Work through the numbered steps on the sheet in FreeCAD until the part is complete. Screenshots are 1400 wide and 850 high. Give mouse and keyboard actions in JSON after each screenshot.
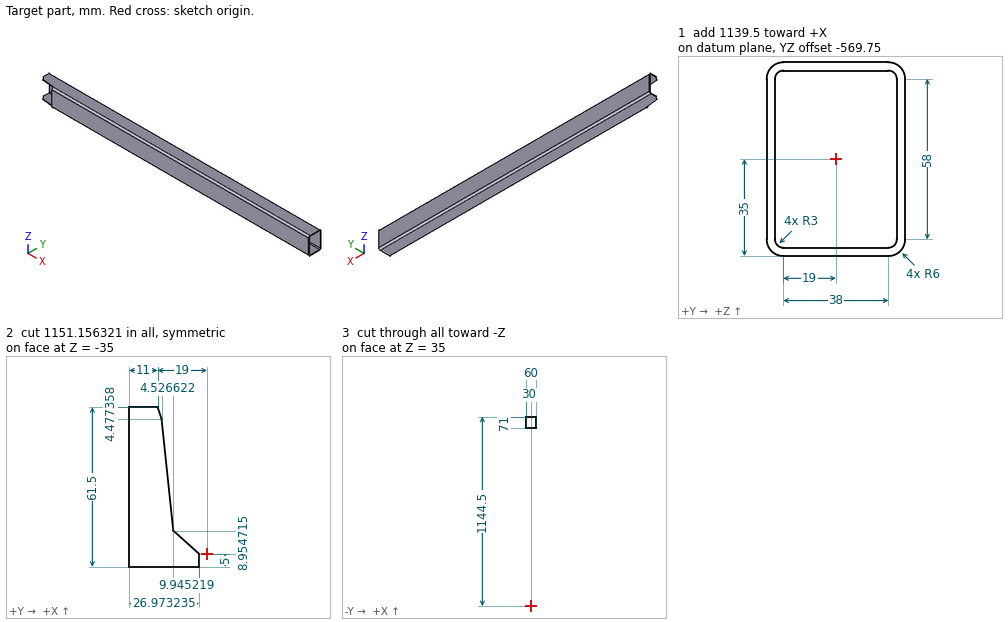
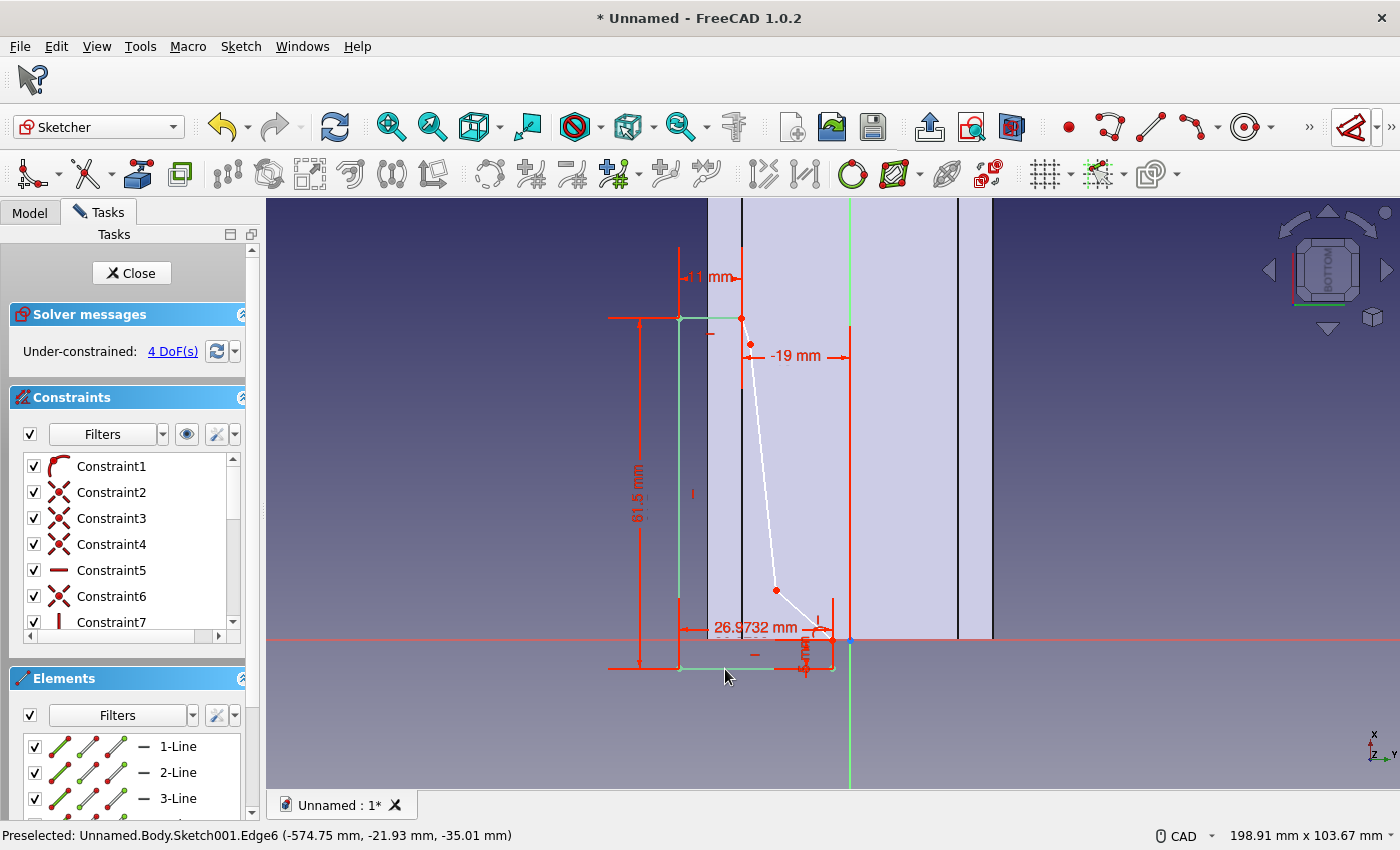
{"action": "left_click", "coordinate": [776, 590]}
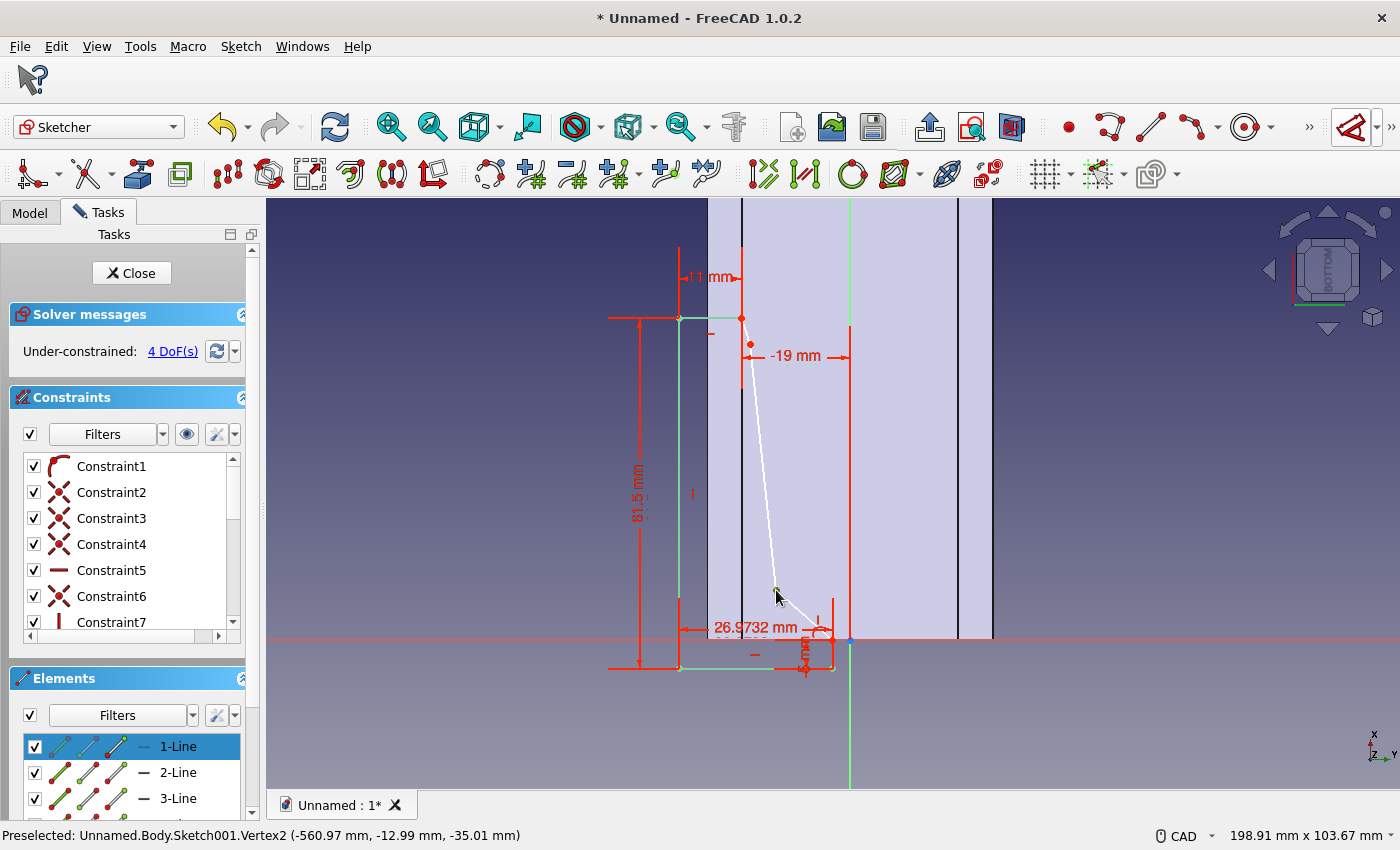
{"action": "key", "text": "i"}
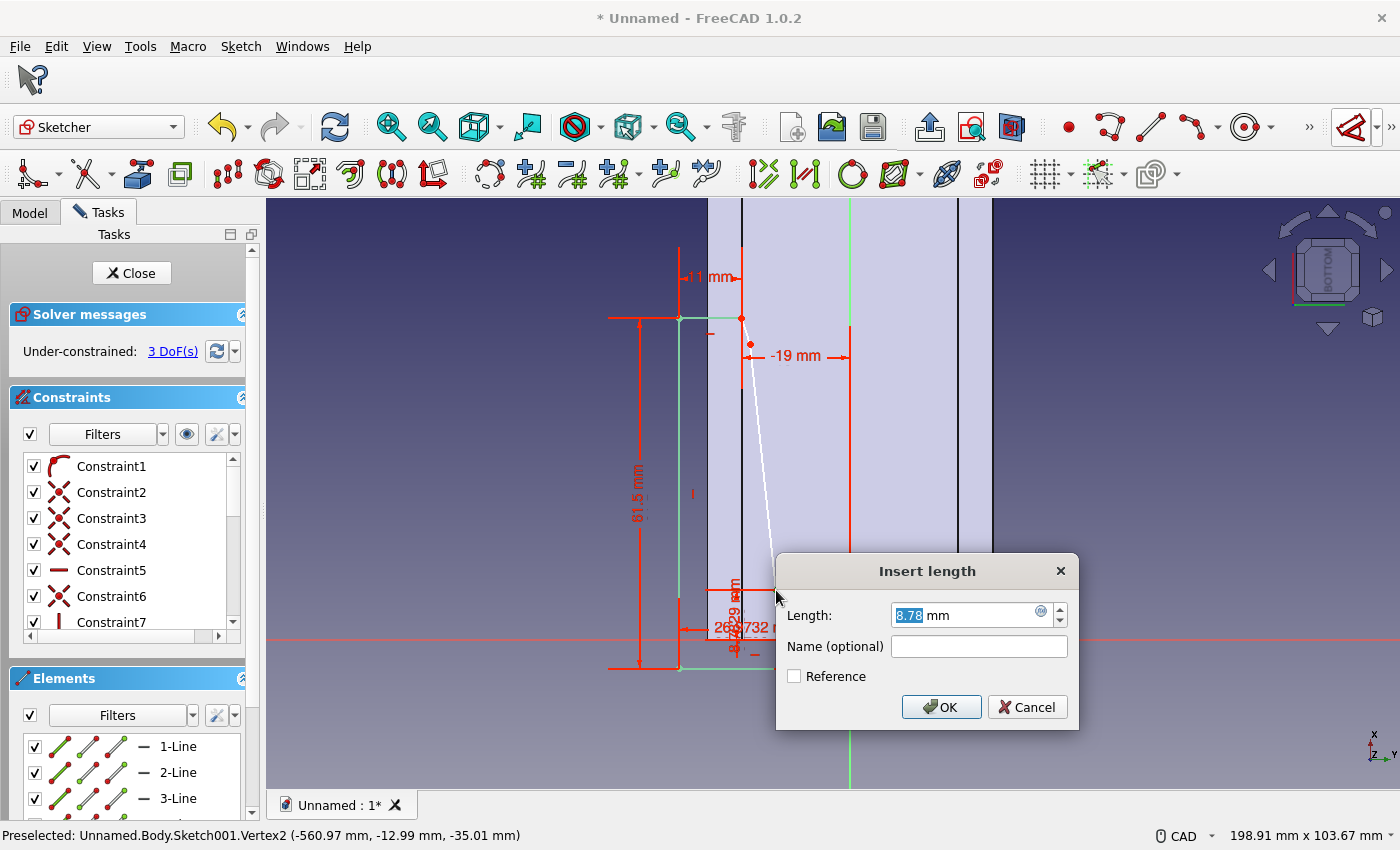
{"action": "type", "text": "8.954715"}
{"action": "key", "text": "Return"}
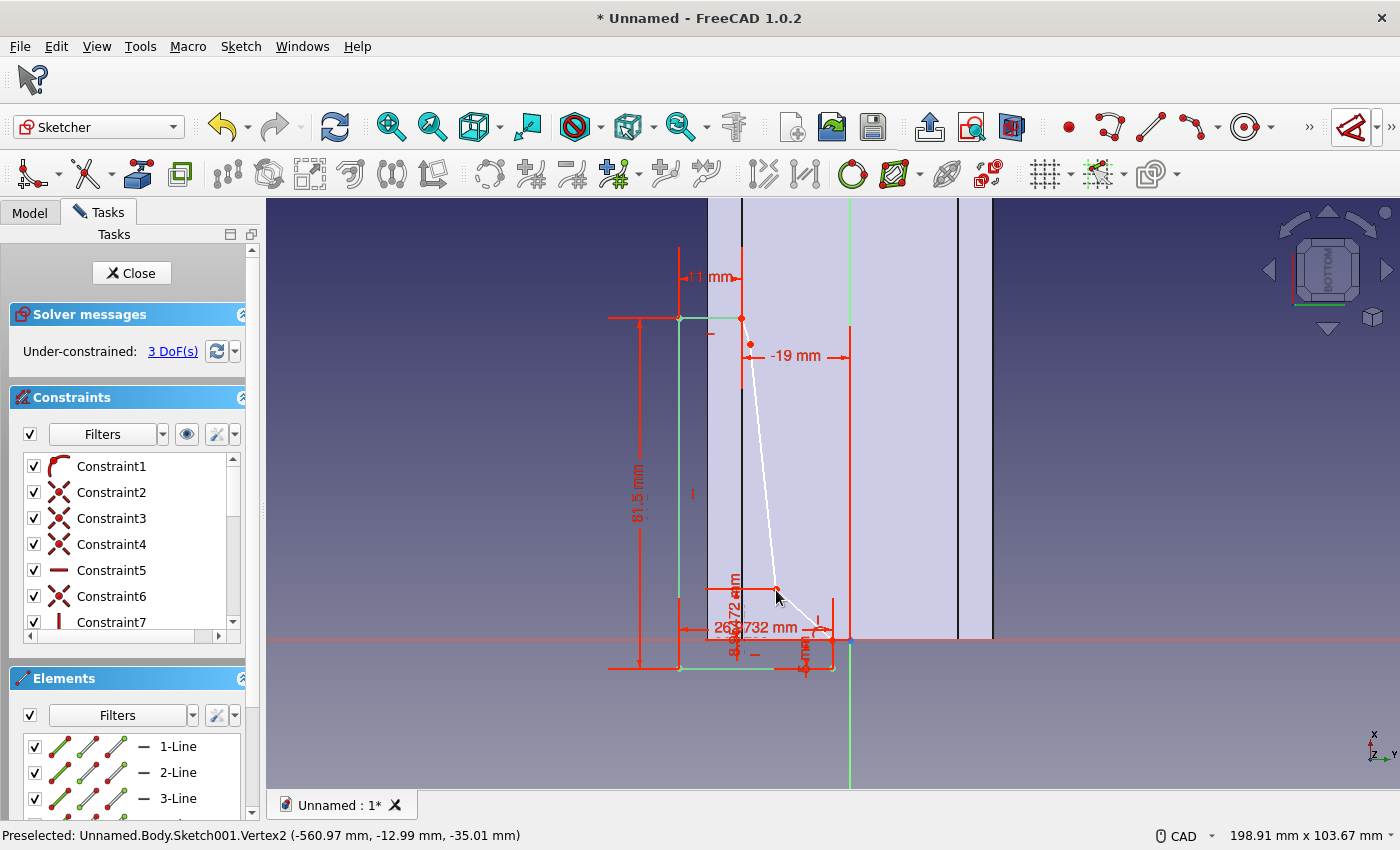
{"action": "left_click", "coordinate": [793, 605]}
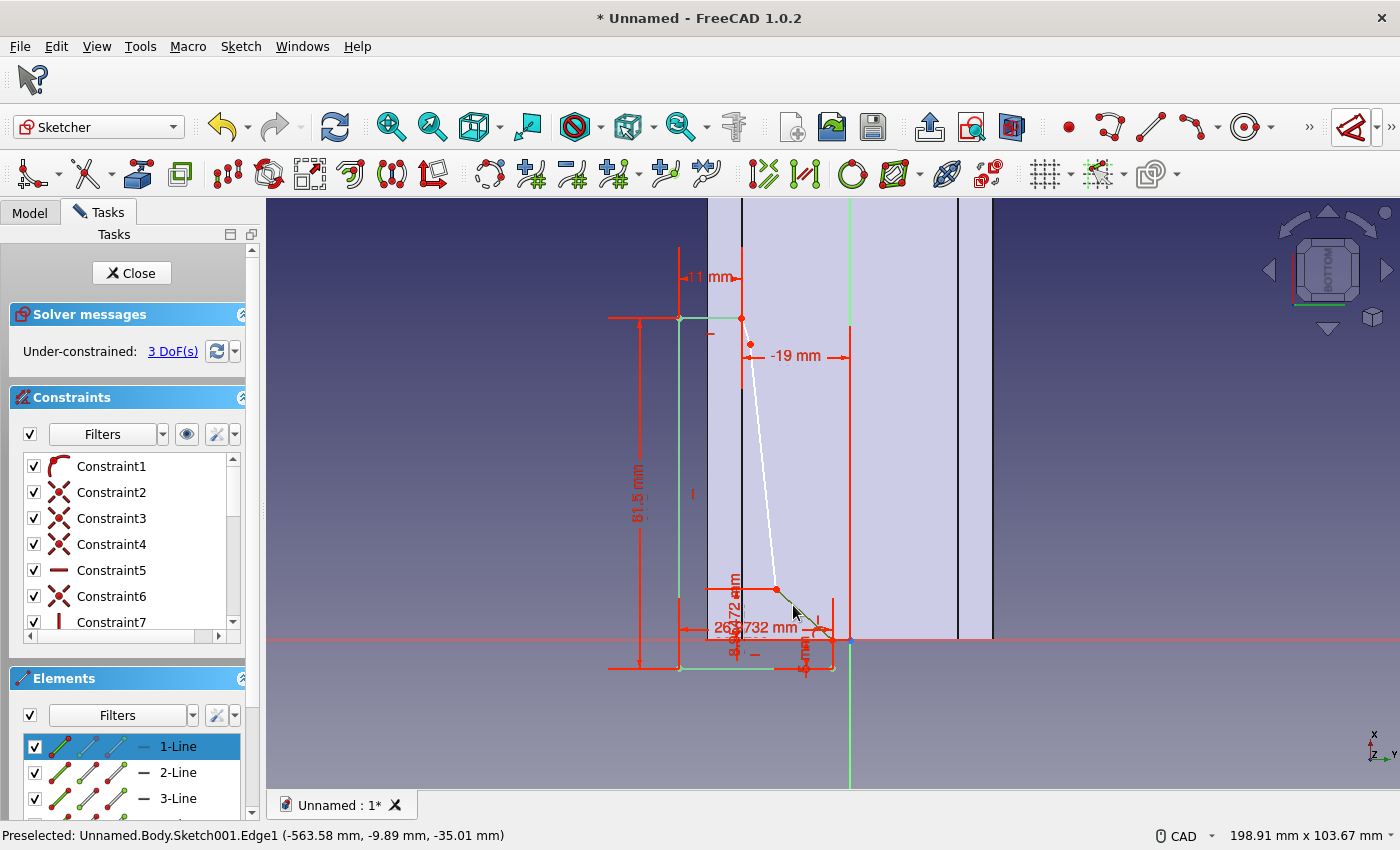
{"action": "left_click", "coordinate": [1376, 128]}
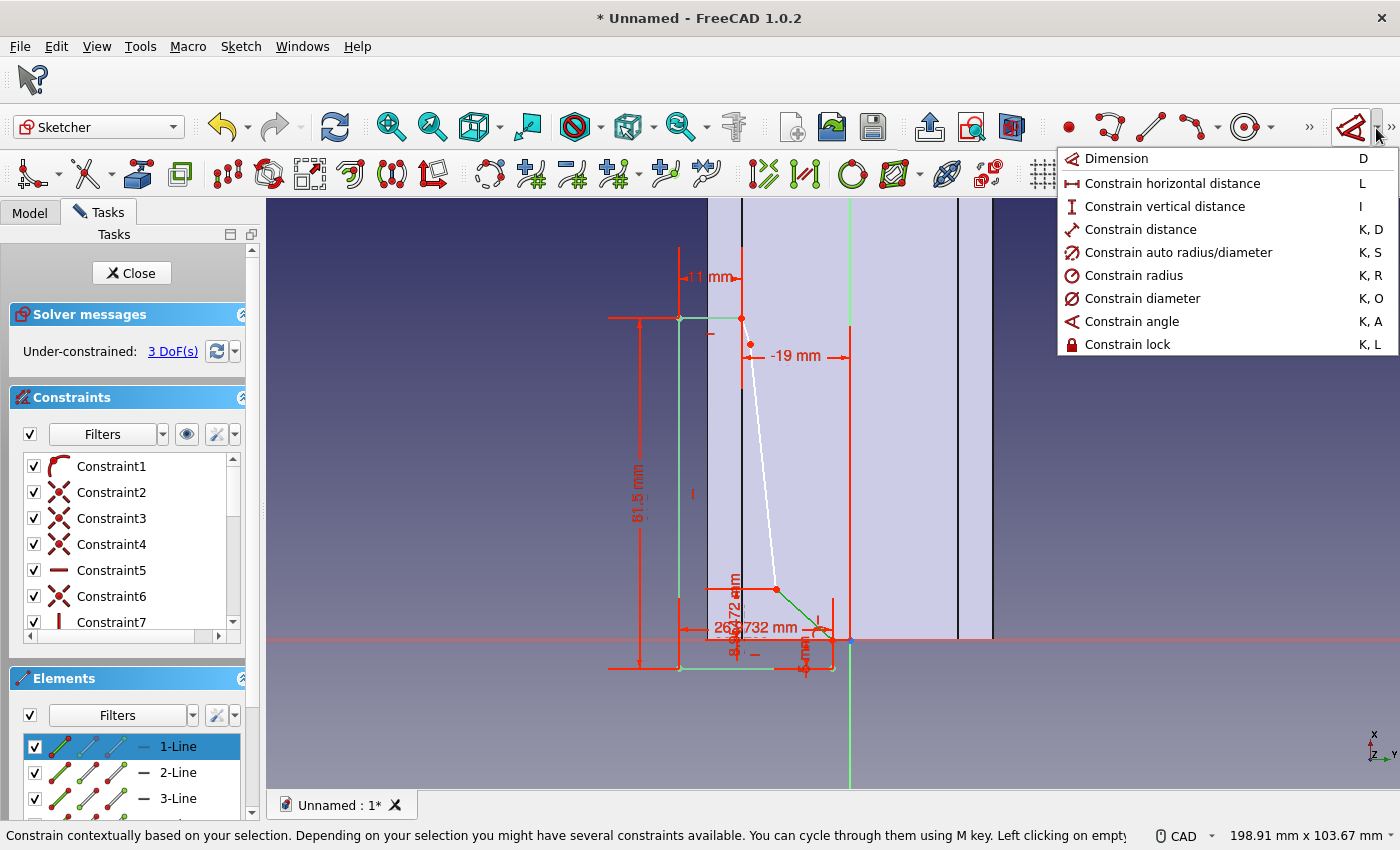
{"action": "left_click", "coordinate": [1228, 184]}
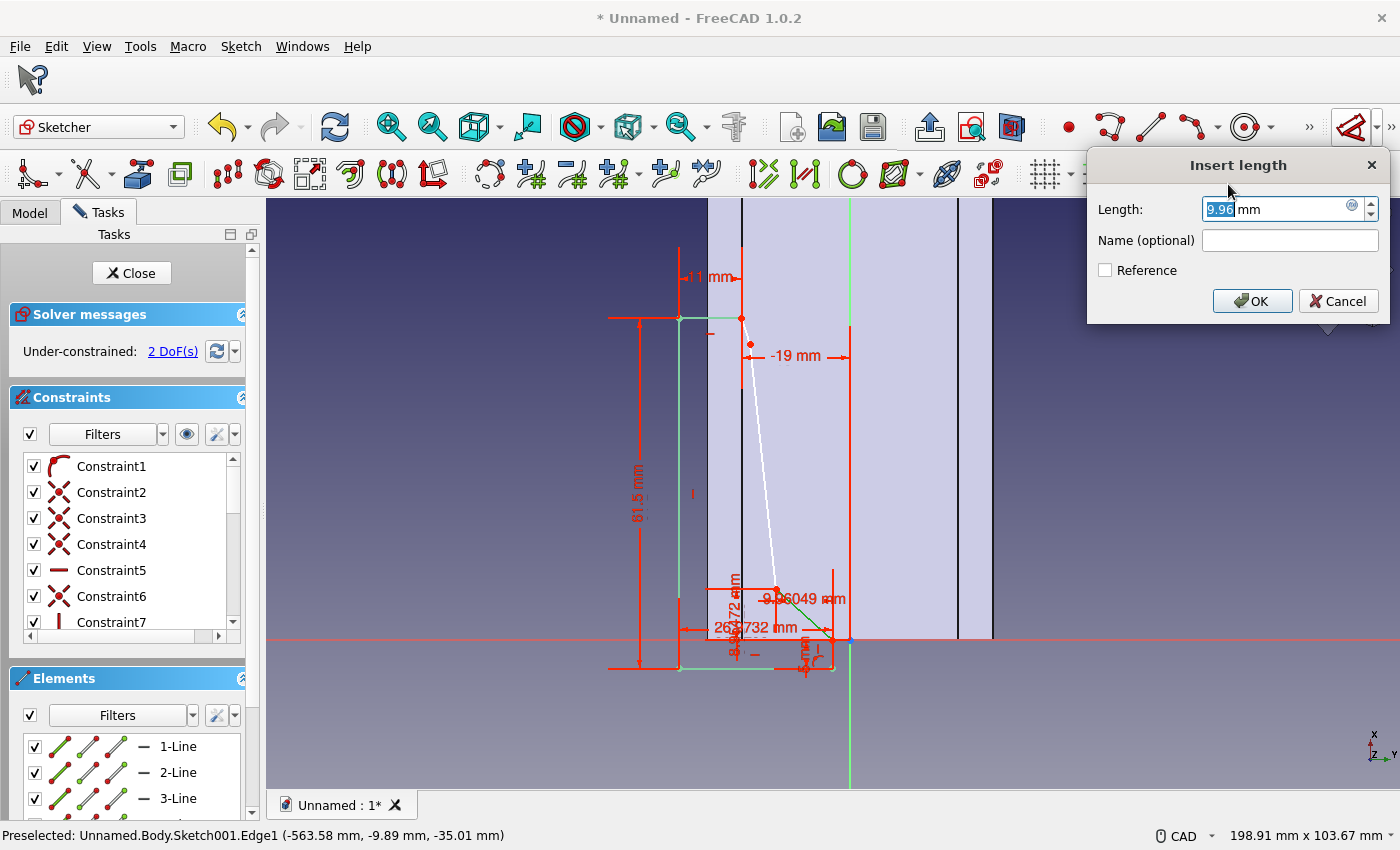
{"action": "type", "text": "9.945219"}
{"action": "key", "text": "Return"}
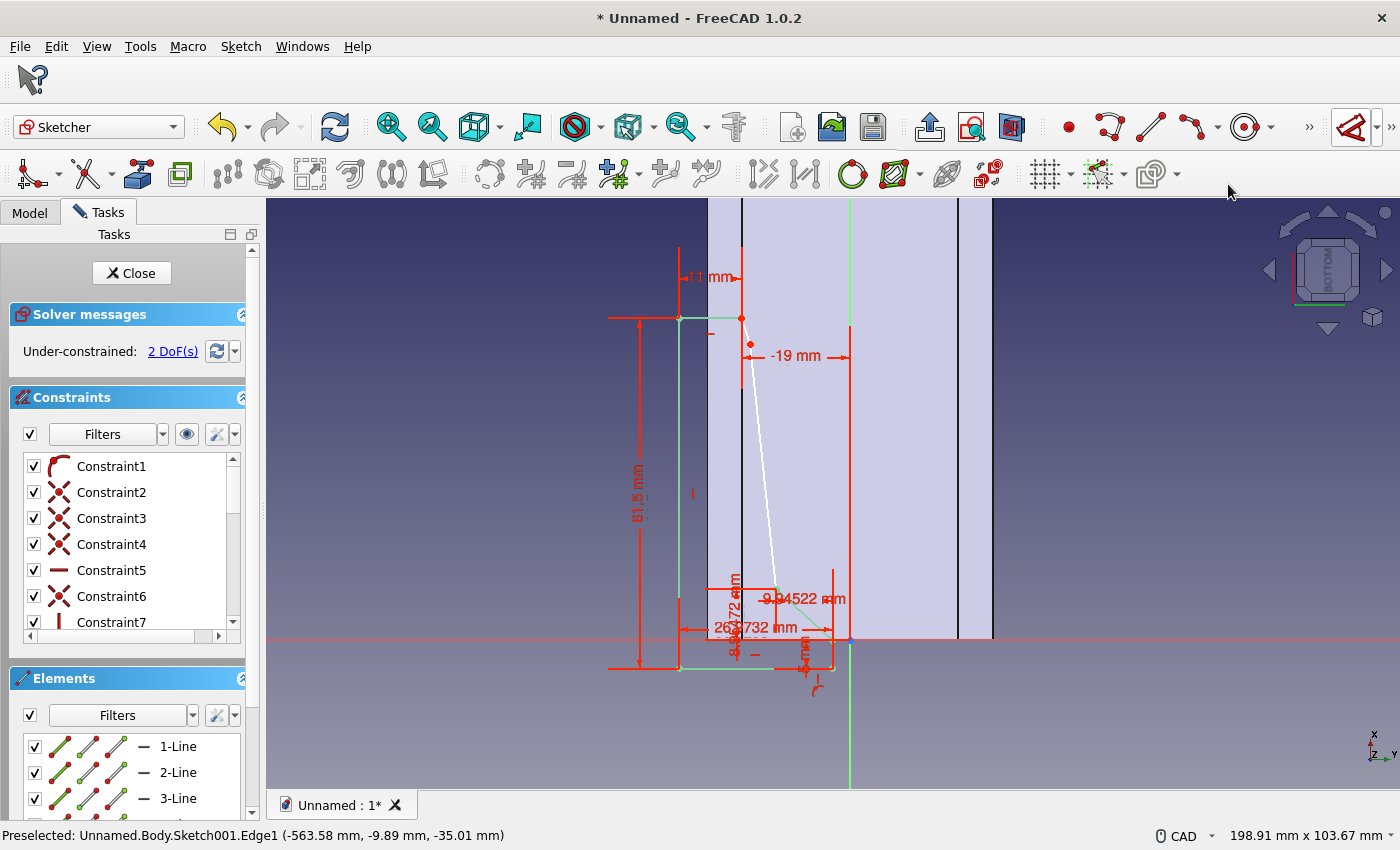
{"action": "scroll", "coordinate": [768, 516], "scroll_direction": "up", "scroll_amount": 3}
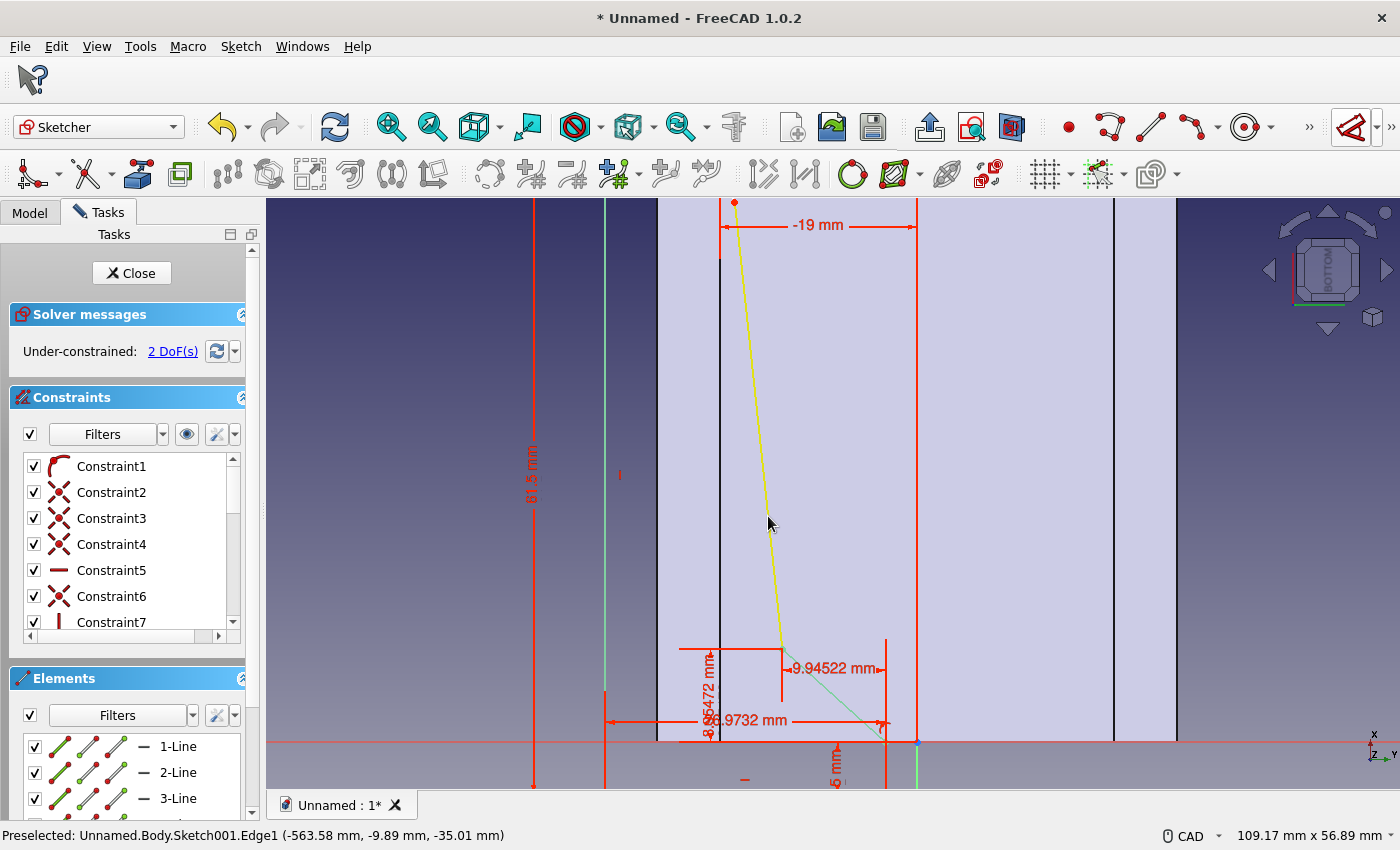
{"action": "left_click", "coordinate": [768, 515]}